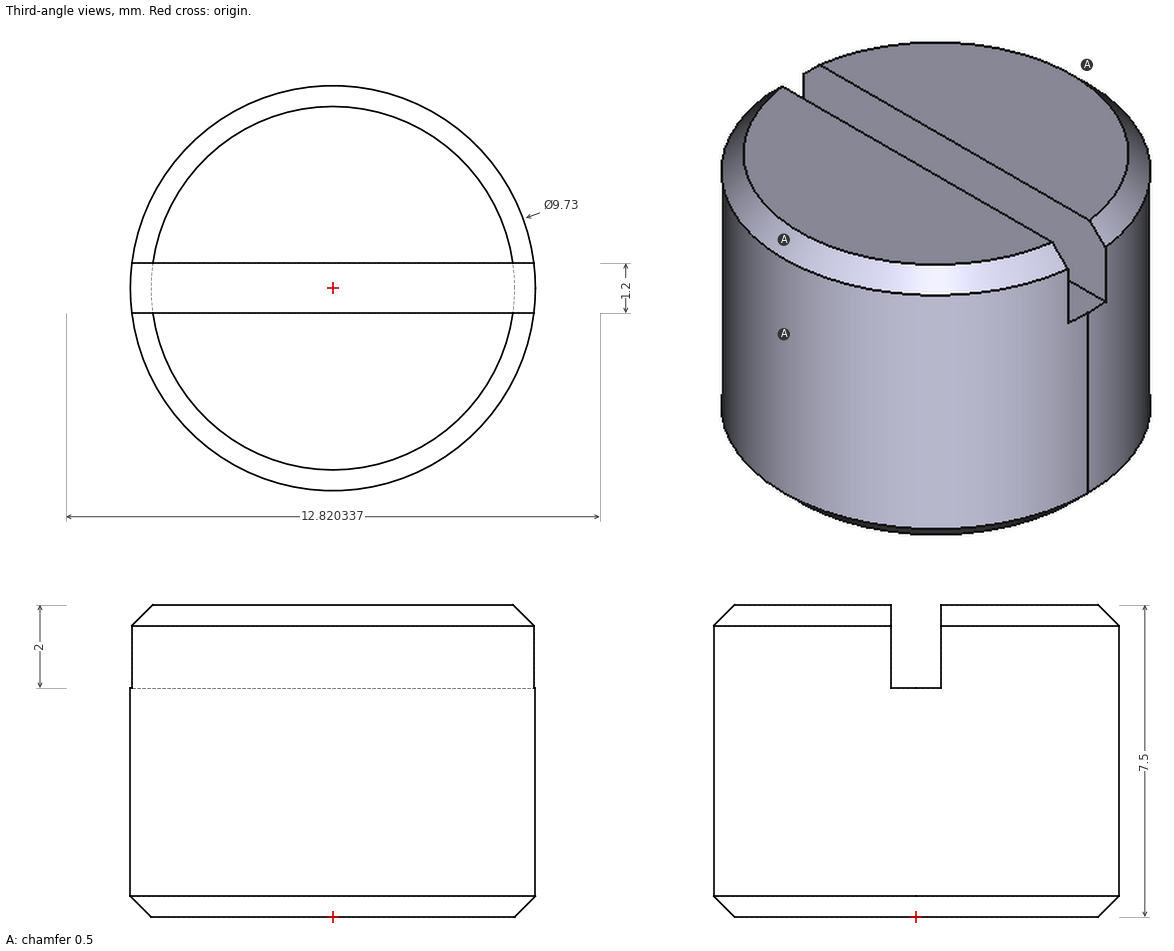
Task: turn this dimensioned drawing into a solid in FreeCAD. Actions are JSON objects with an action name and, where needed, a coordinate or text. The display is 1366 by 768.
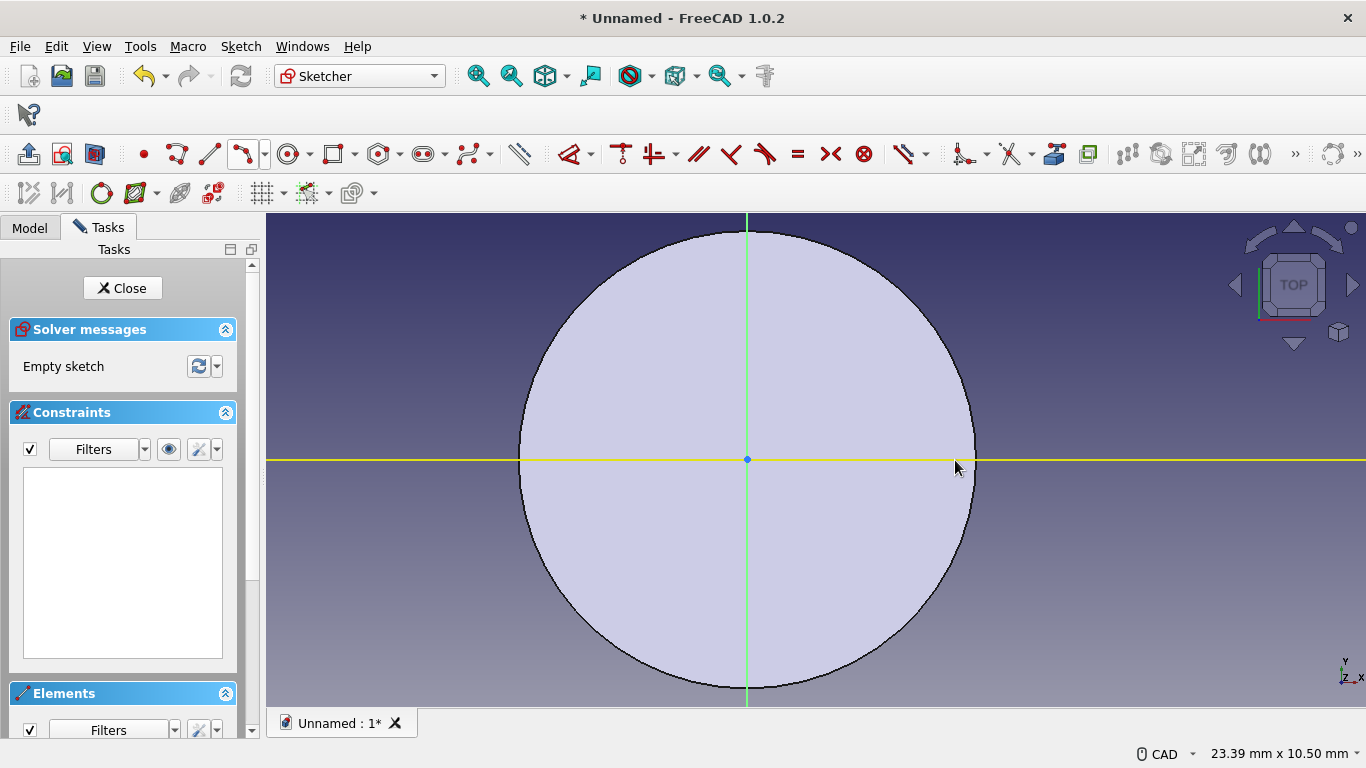
{"action": "left_click", "coordinate": [354, 154]}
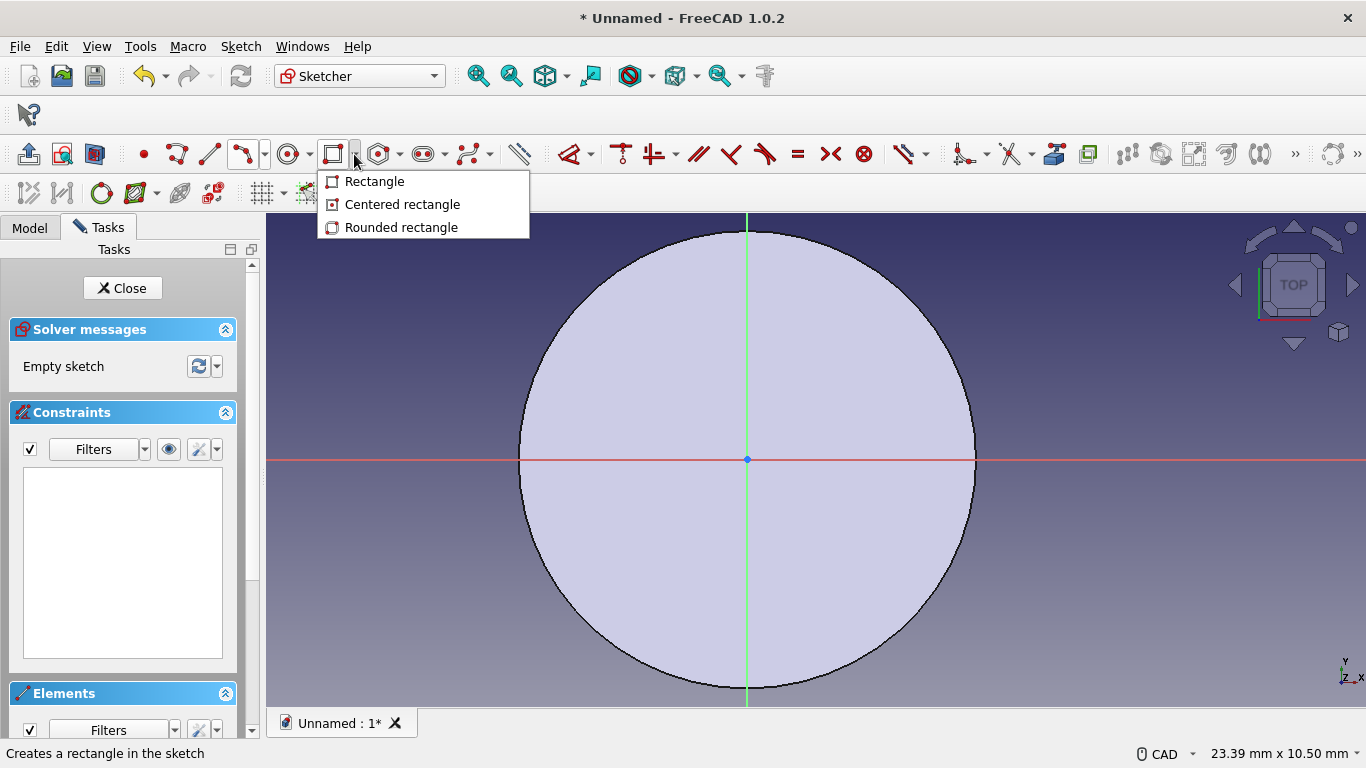
{"action": "left_click", "coordinate": [424, 204]}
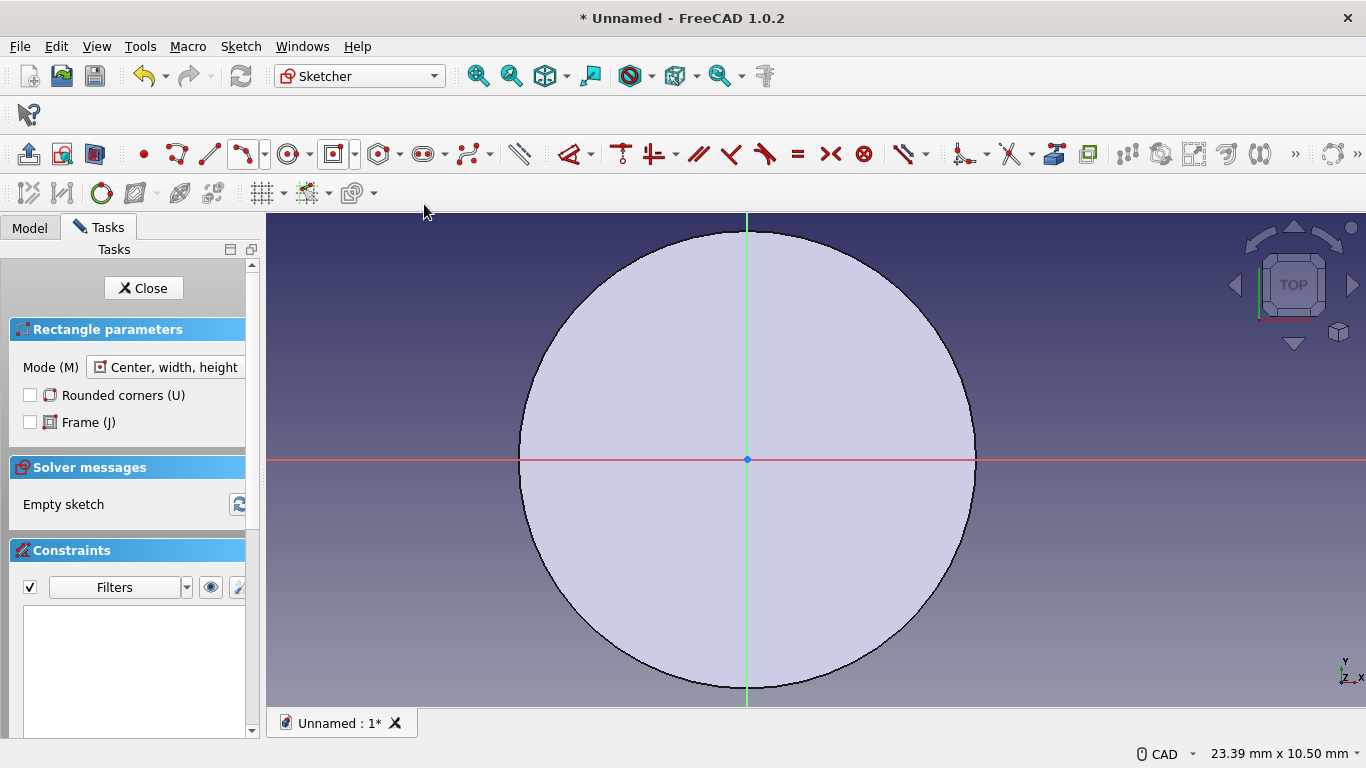
{"action": "left_click", "coordinate": [747, 460]}
{"action": "left_click", "coordinate": [1049, 432]}
{"action": "key", "text": "Escape"}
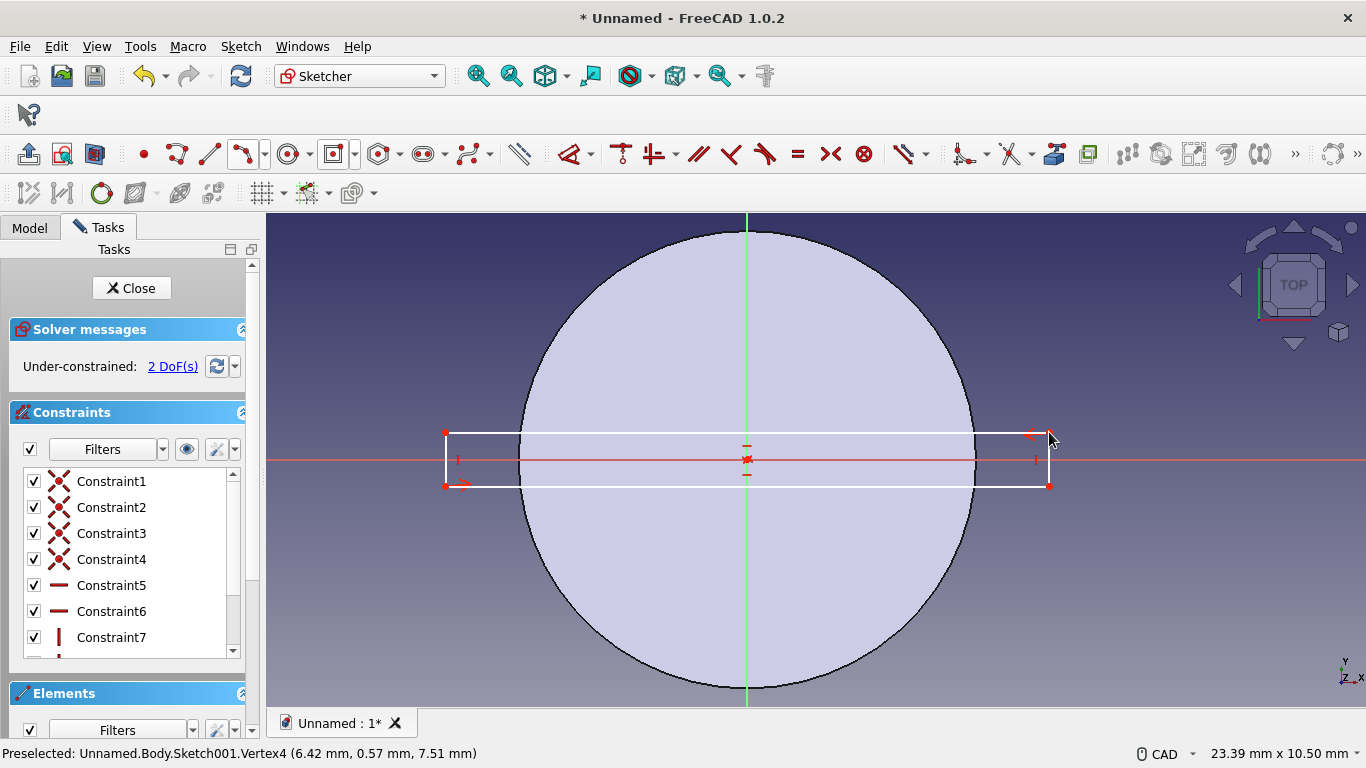
{"action": "left_click", "coordinate": [568, 154]}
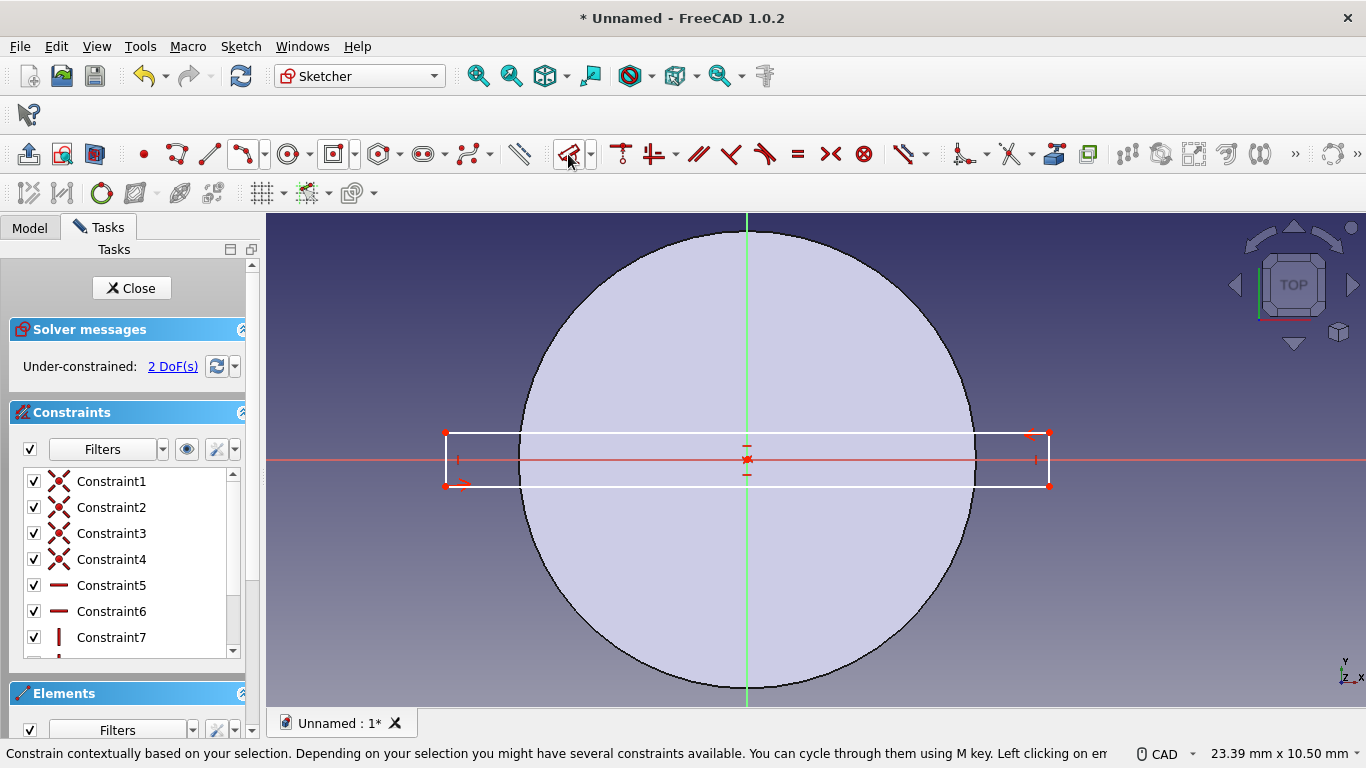
{"action": "scroll", "coordinate": [1049, 470], "scroll_direction": "up", "scroll_amount": 2}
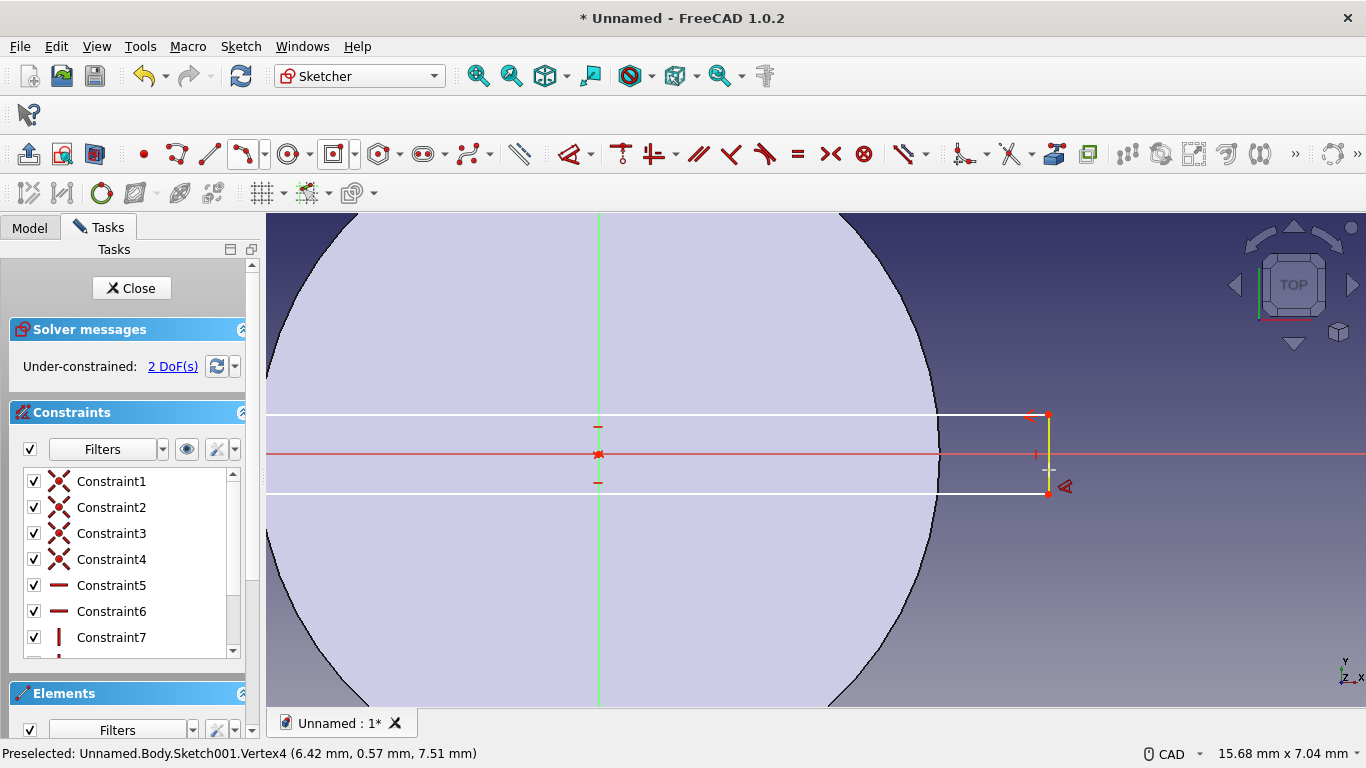
{"action": "left_click", "coordinate": [1049, 470]}
{"action": "left_click", "coordinate": [1083, 436]}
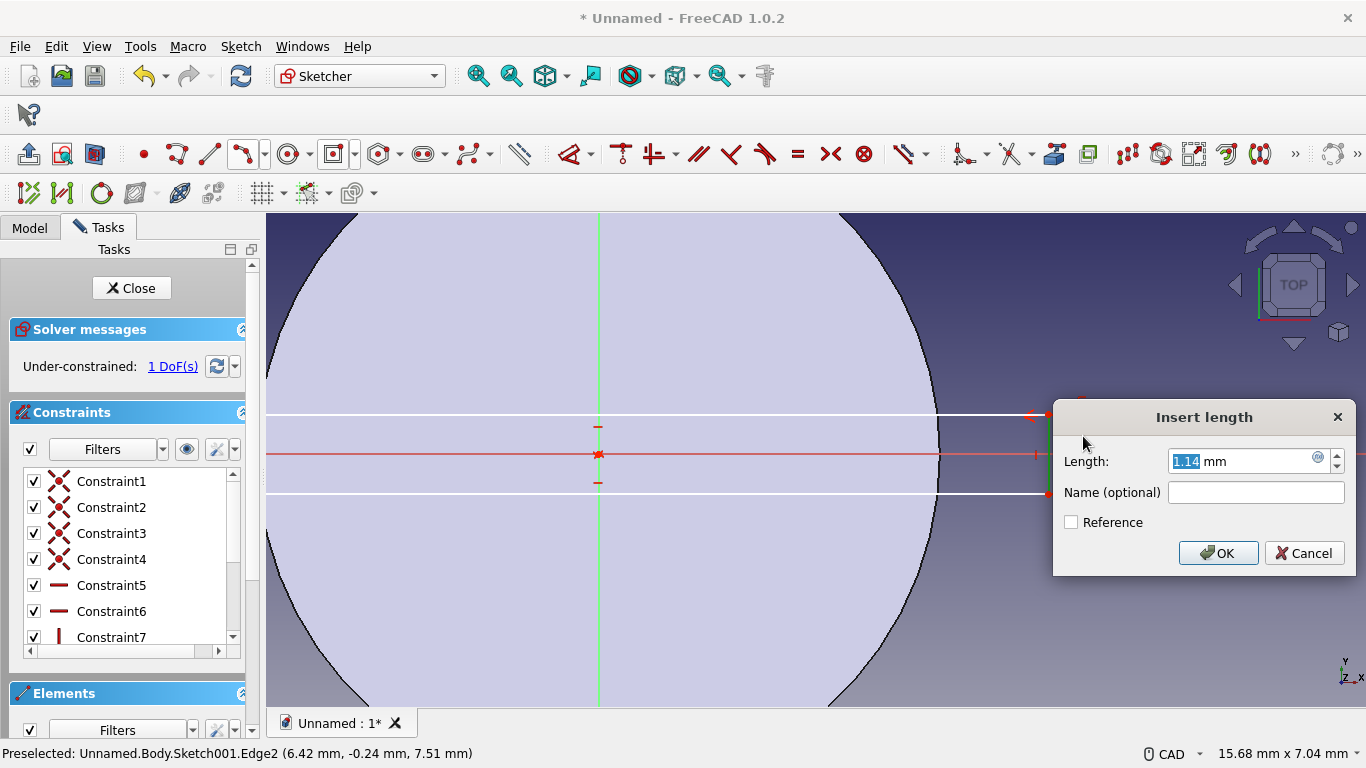
{"action": "type", "text": "1.2"}
{"action": "key", "text": "Return"}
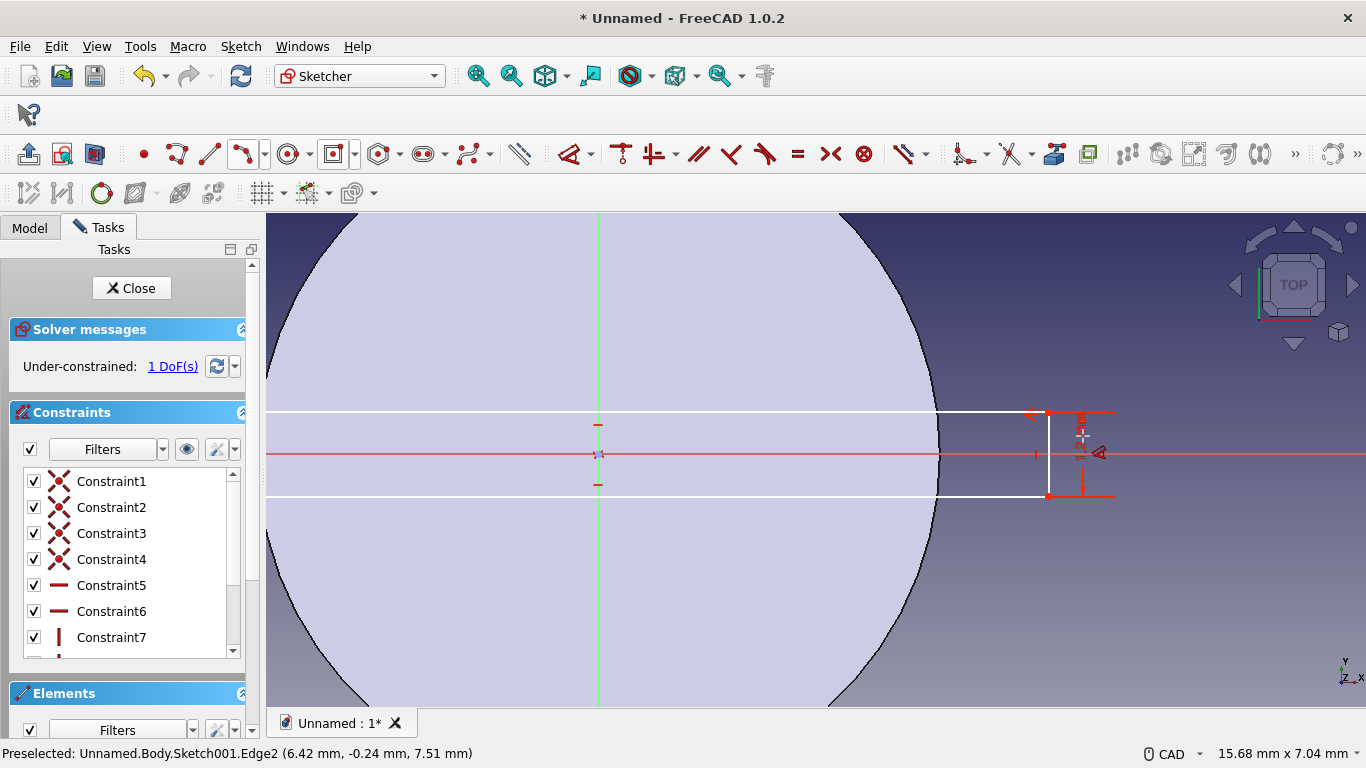
{"action": "left_click", "coordinate": [419, 497]}
{"action": "left_click", "coordinate": [671, 531]}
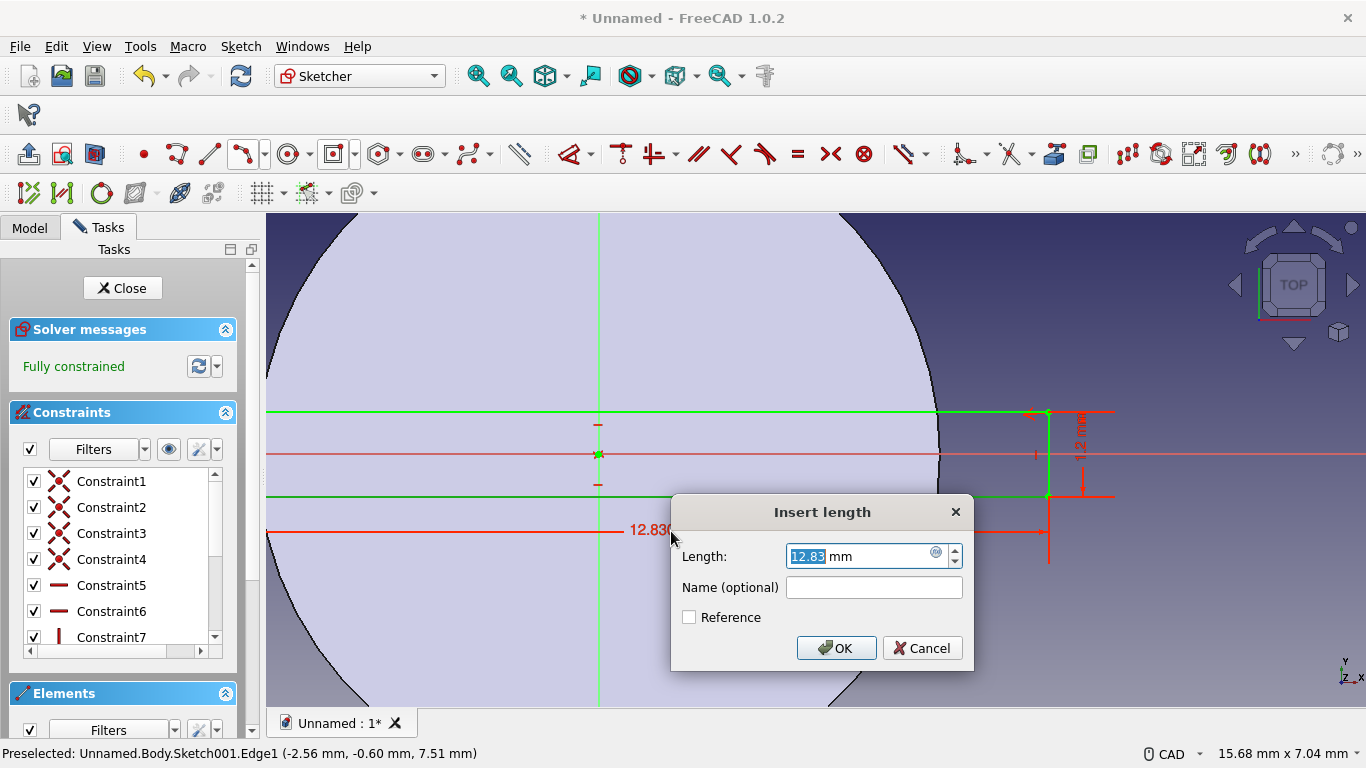
{"action": "type", "text": "12.820337"}
{"action": "key", "text": "Return"}
{"action": "key", "text": "Escape"}